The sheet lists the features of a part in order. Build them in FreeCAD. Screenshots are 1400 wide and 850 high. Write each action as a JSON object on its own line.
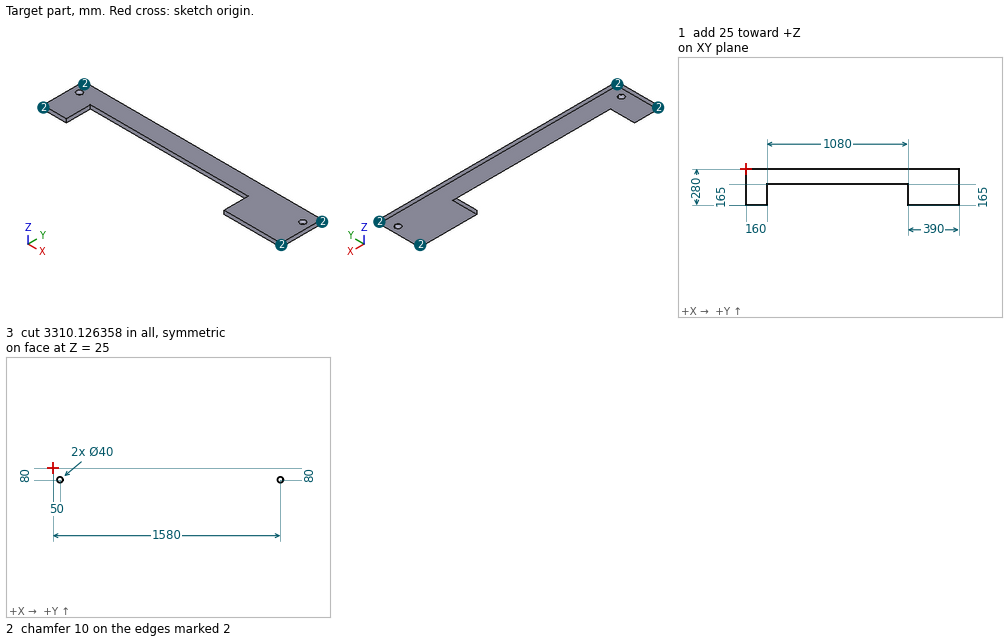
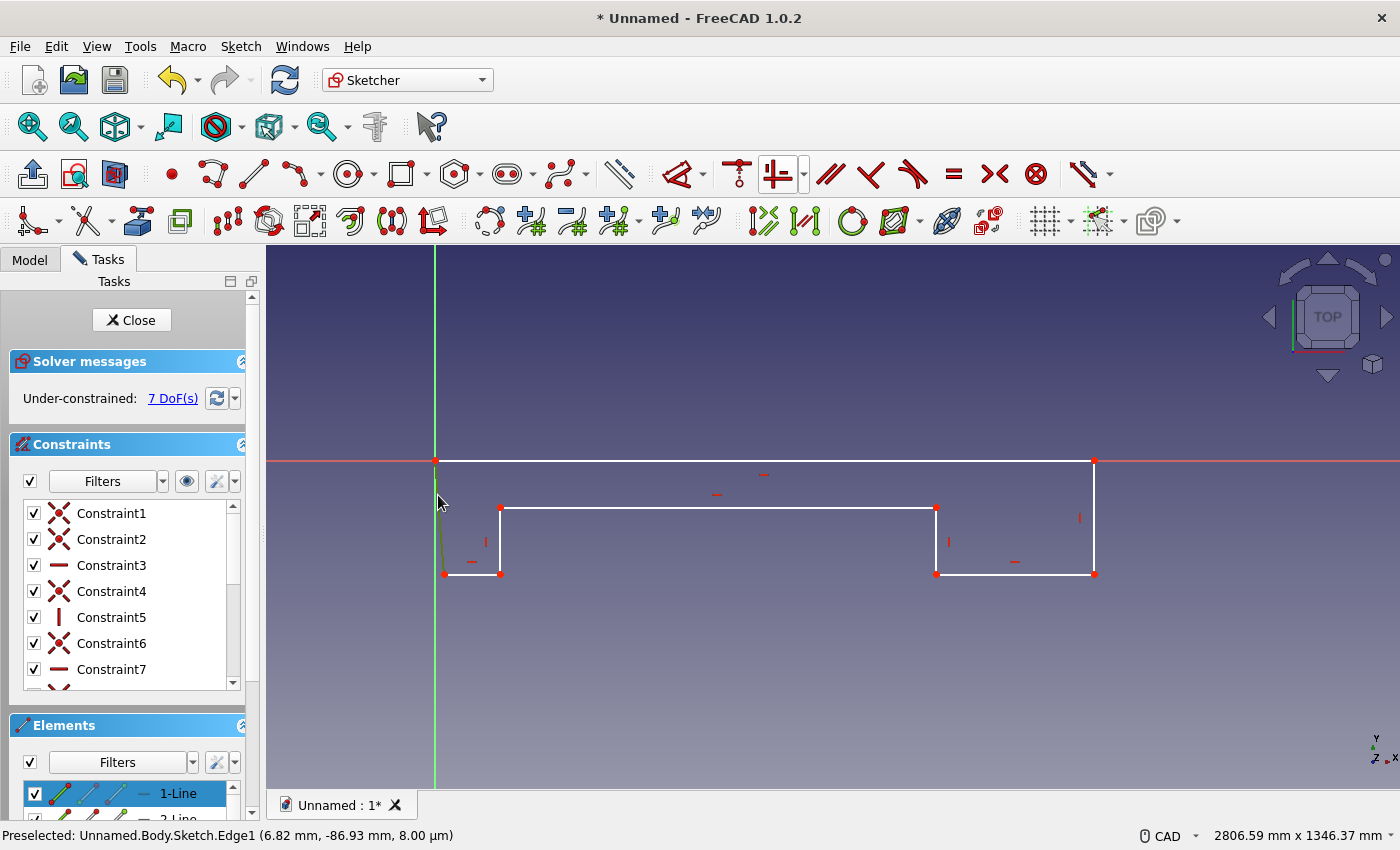
{"action": "key", "text": "v"}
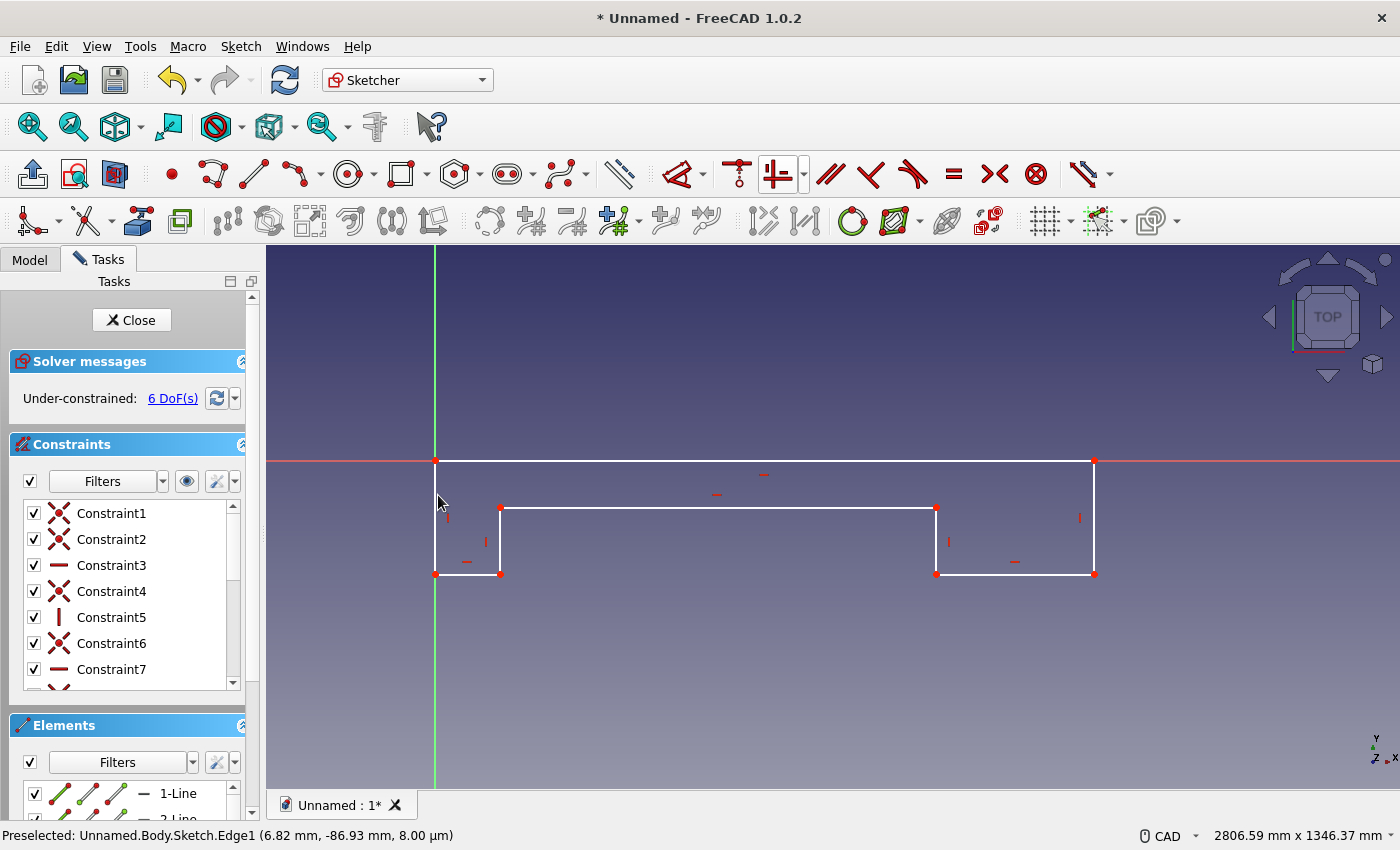
{"action": "key", "text": "d"}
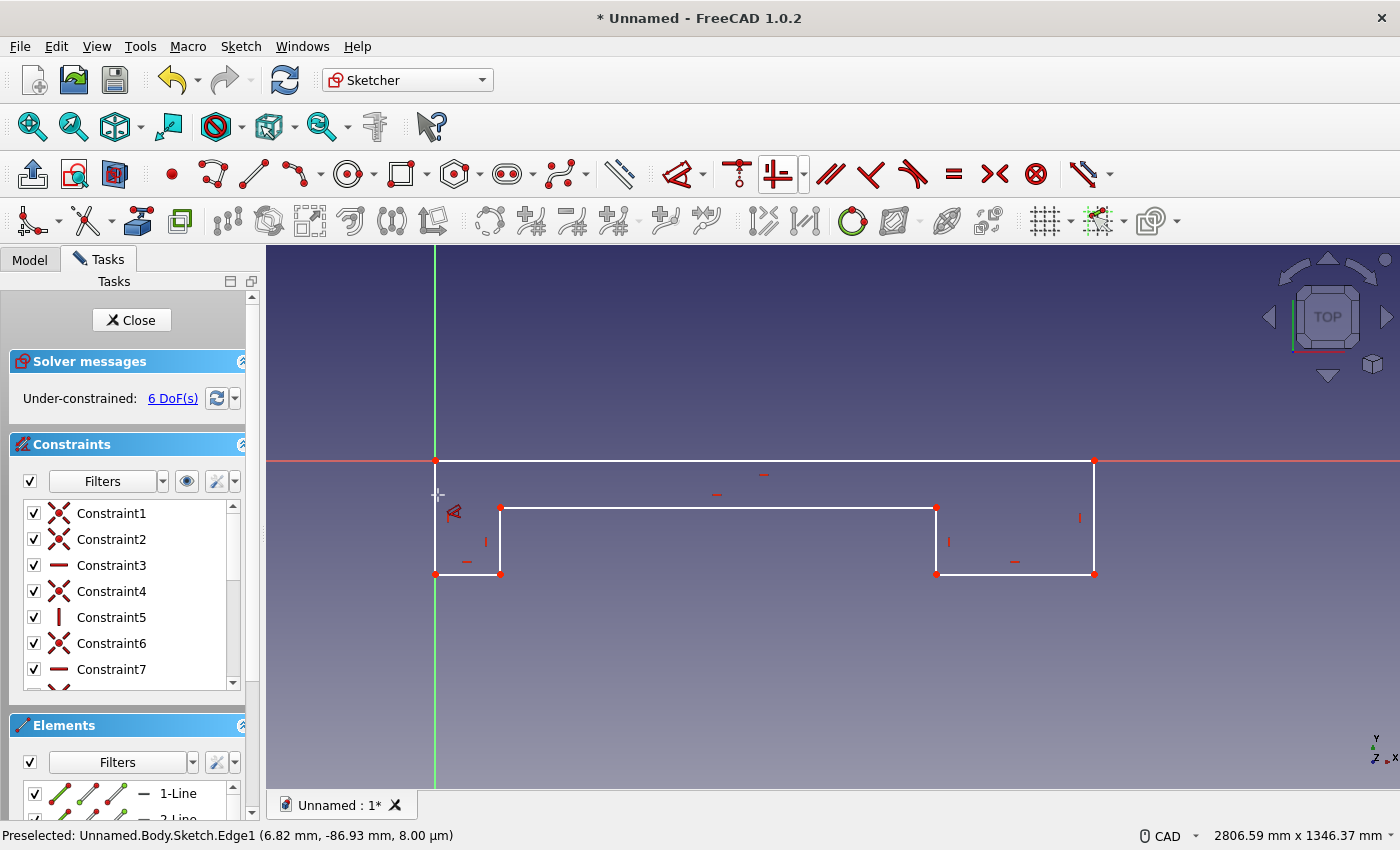
{"action": "left_click", "coordinate": [435, 495]}
{"action": "left_click", "coordinate": [401, 518]}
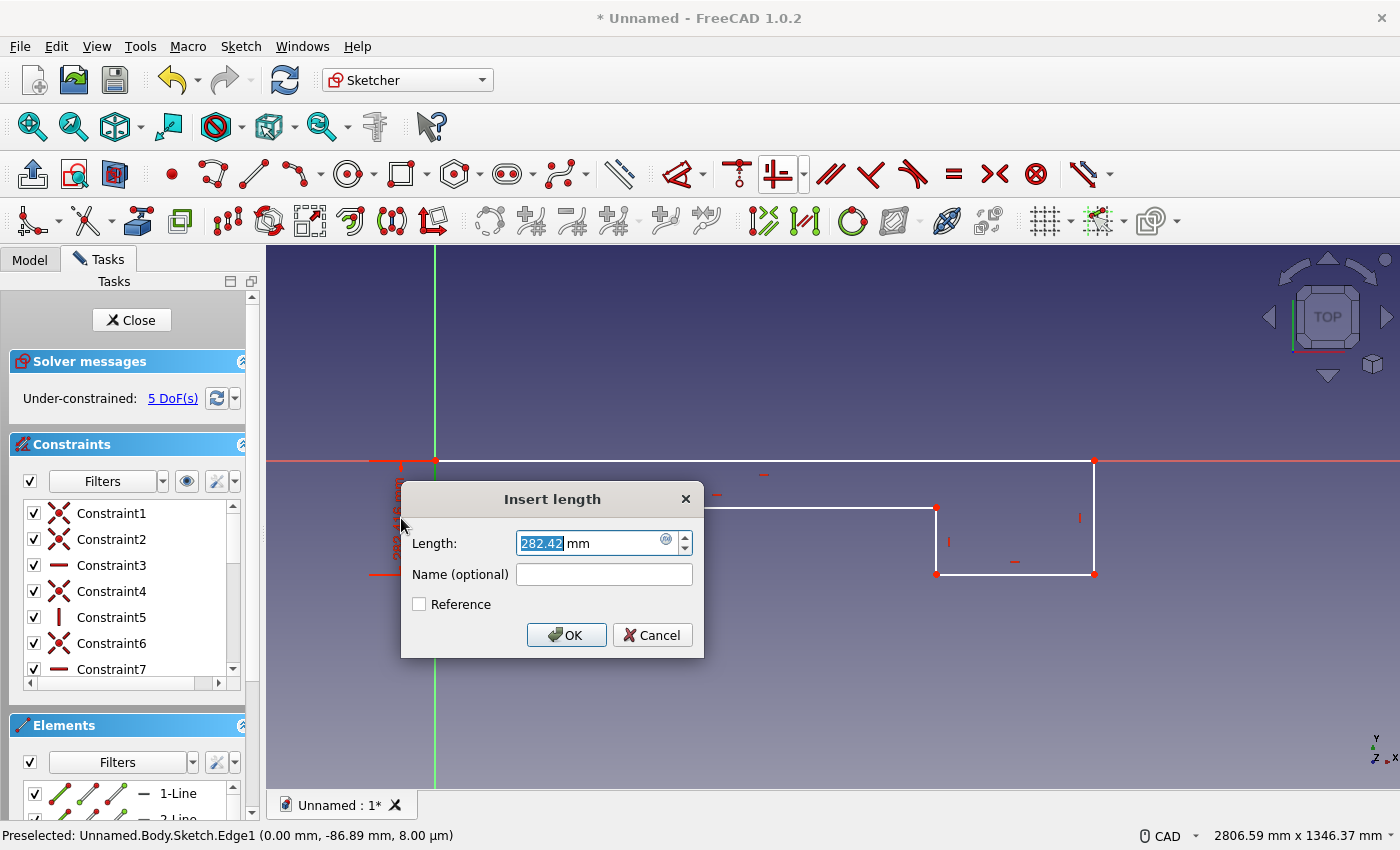
{"action": "type", "text": "280"}
{"action": "key", "text": "Return"}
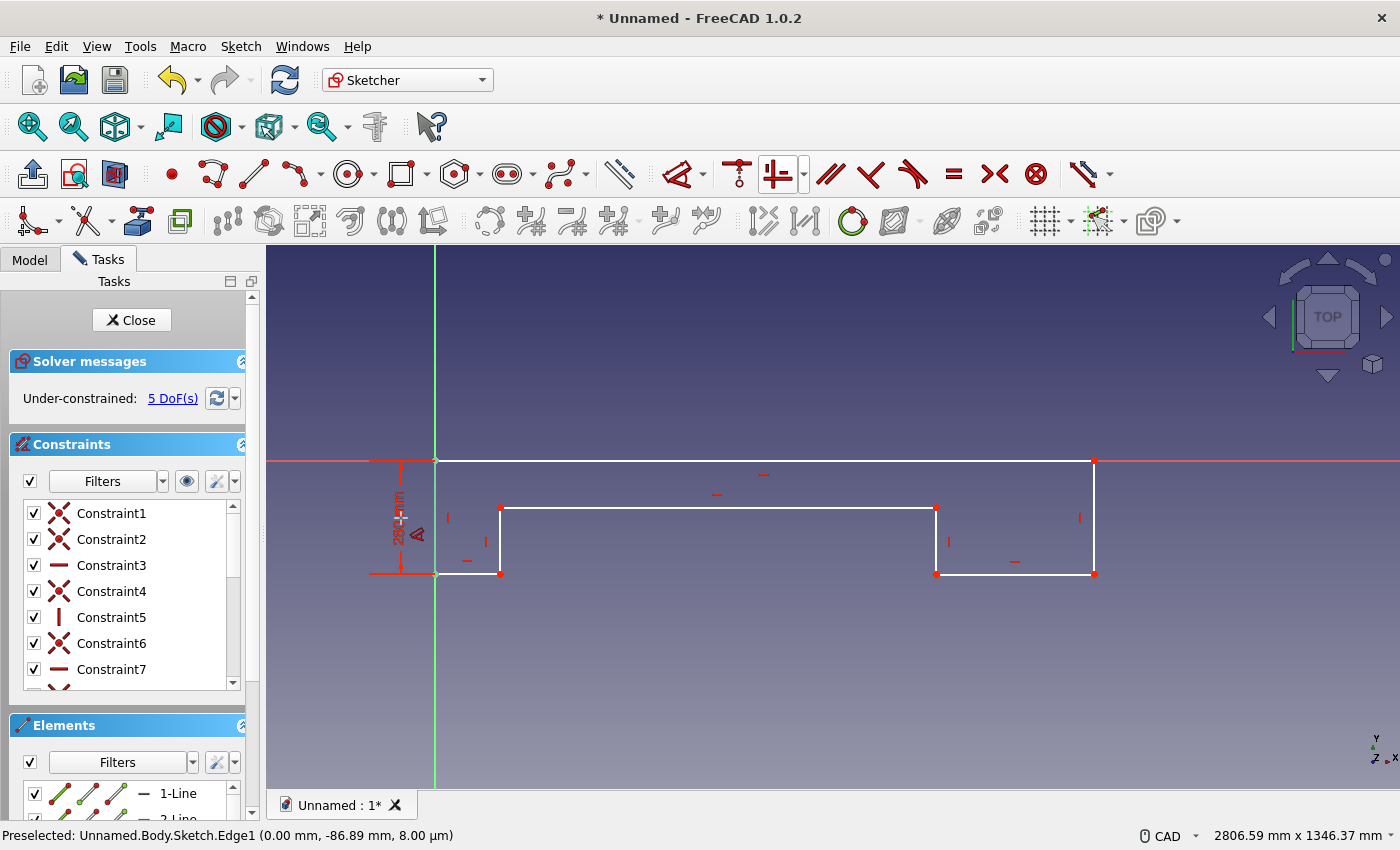
{"action": "left_click", "coordinate": [455, 574]}
{"action": "left_click", "coordinate": [468, 608]}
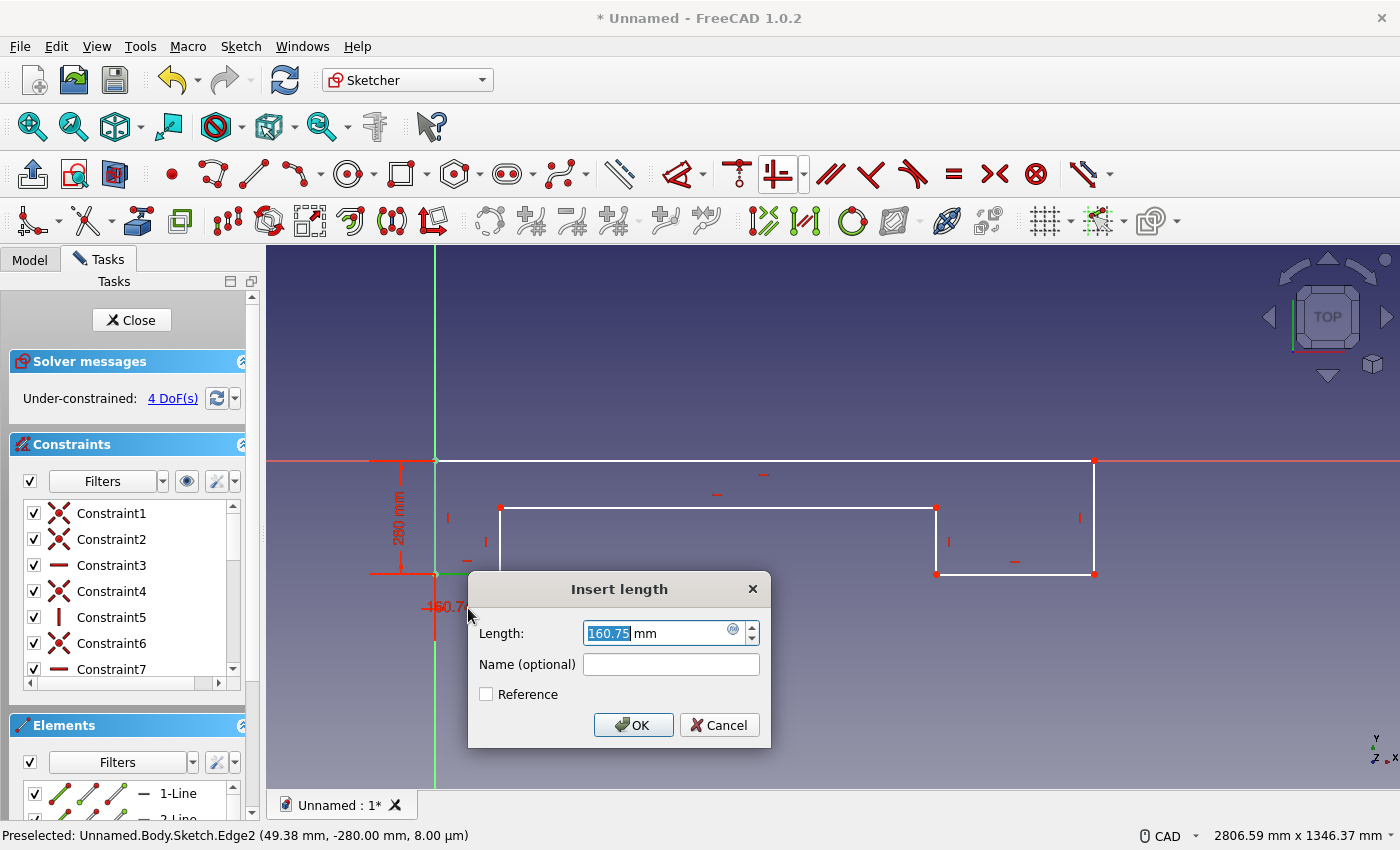
{"action": "type", "text": "160"}
{"action": "key", "text": "Return"}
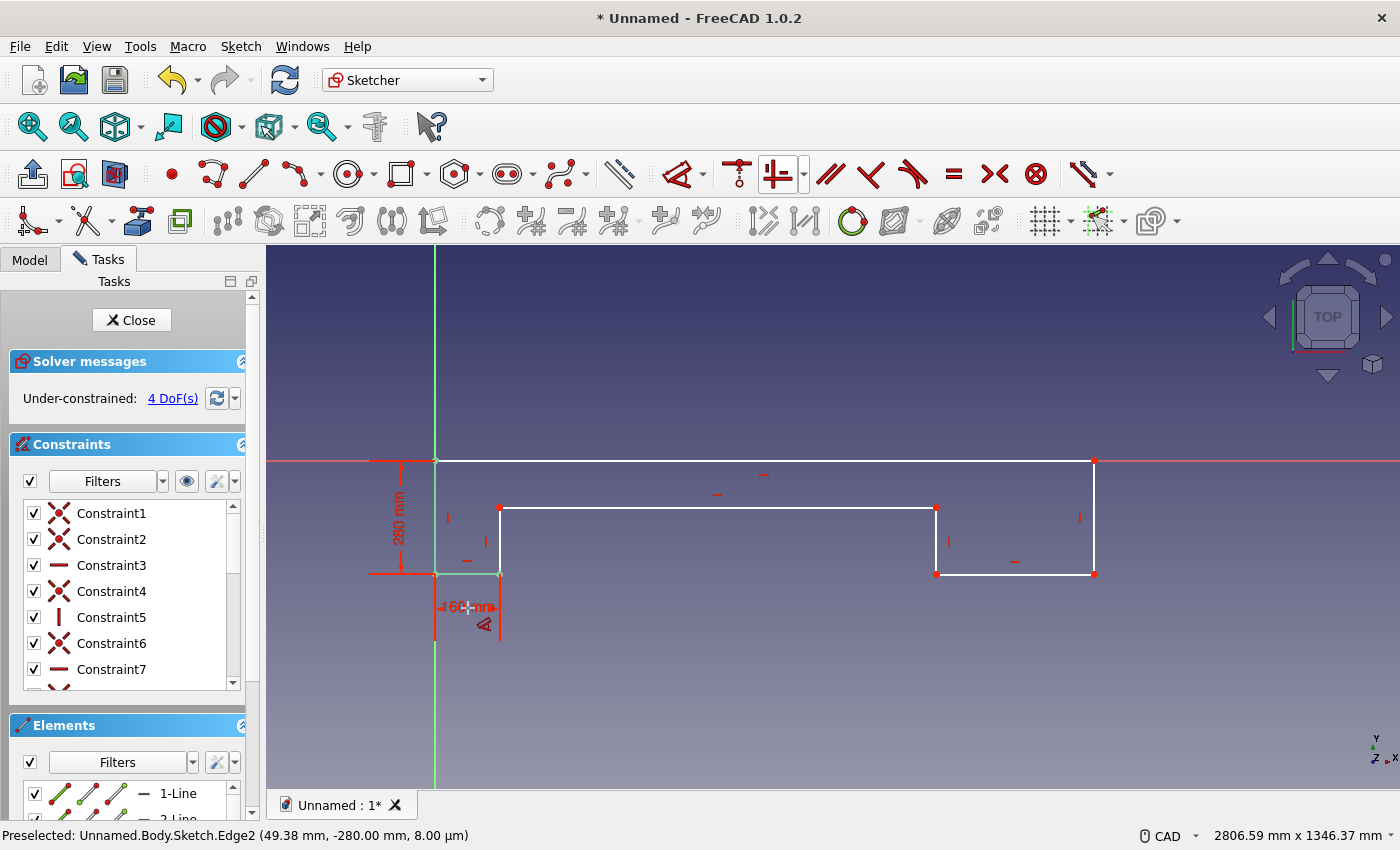
{"action": "left_click", "coordinate": [500, 554]}
{"action": "left_click", "coordinate": [466, 541]}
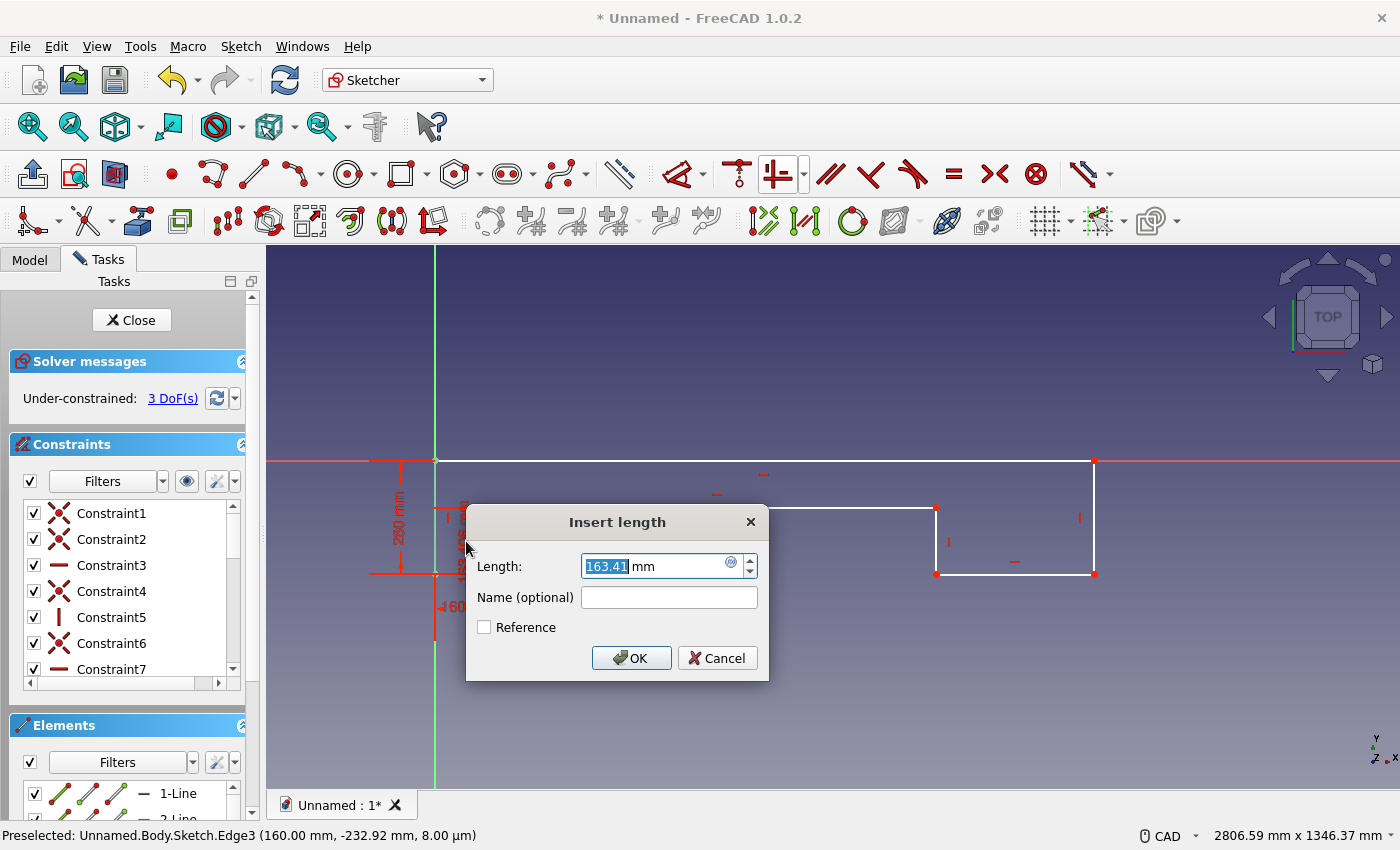
{"action": "type", "text": "165"}
{"action": "key", "text": "Return"}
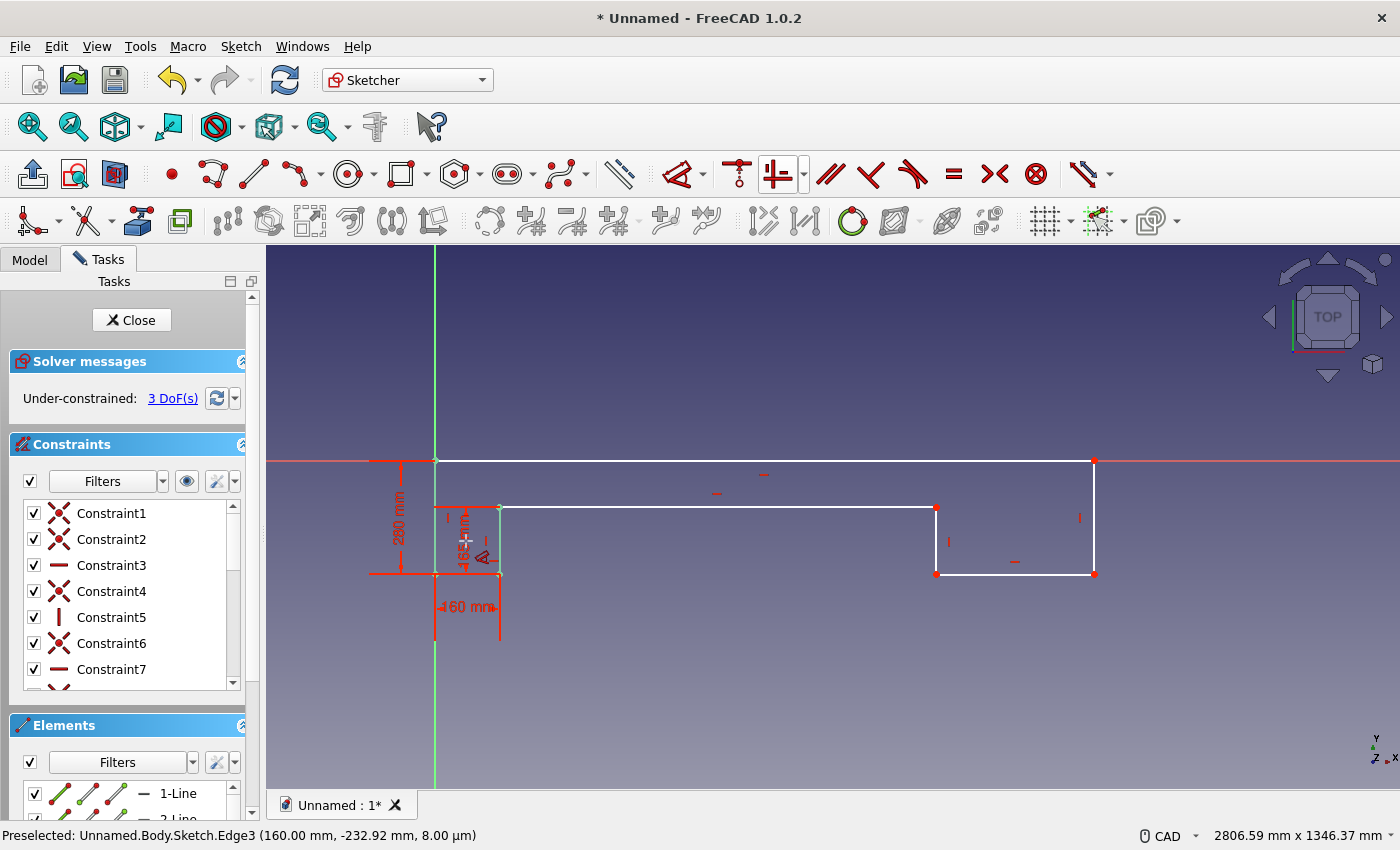
{"action": "left_click", "coordinate": [936, 528]}
{"action": "left_click", "coordinate": [970, 541]}